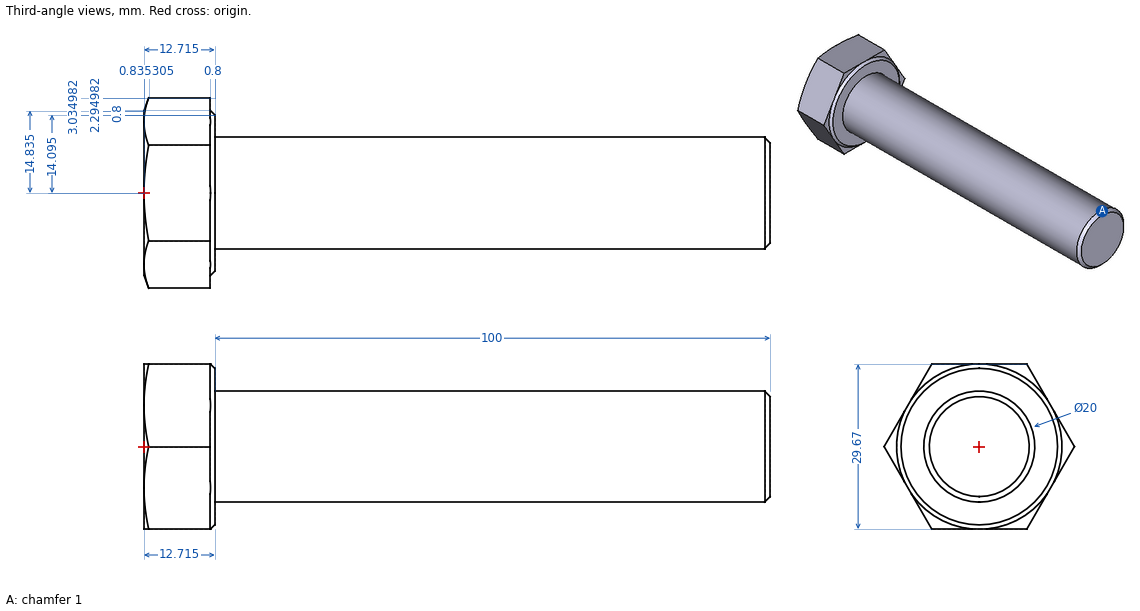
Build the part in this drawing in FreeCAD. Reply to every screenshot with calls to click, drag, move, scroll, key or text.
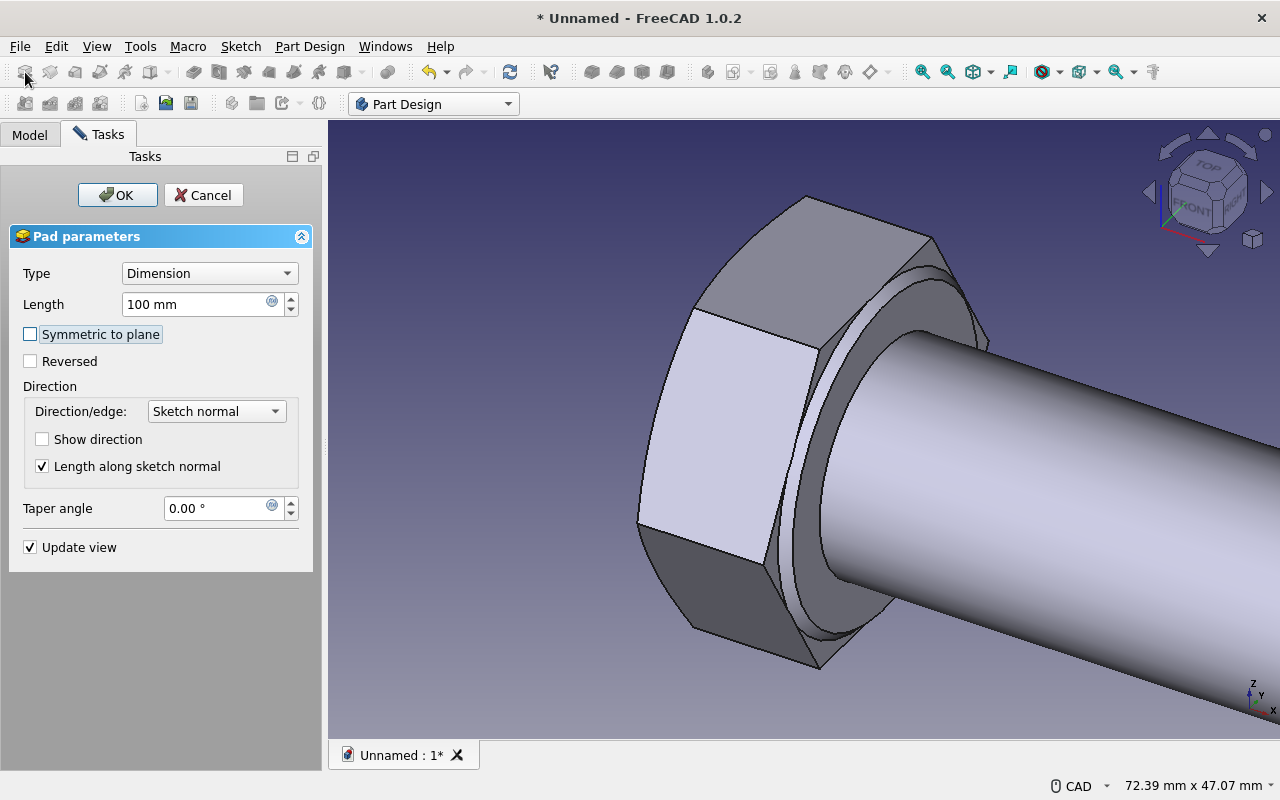
click(118, 195)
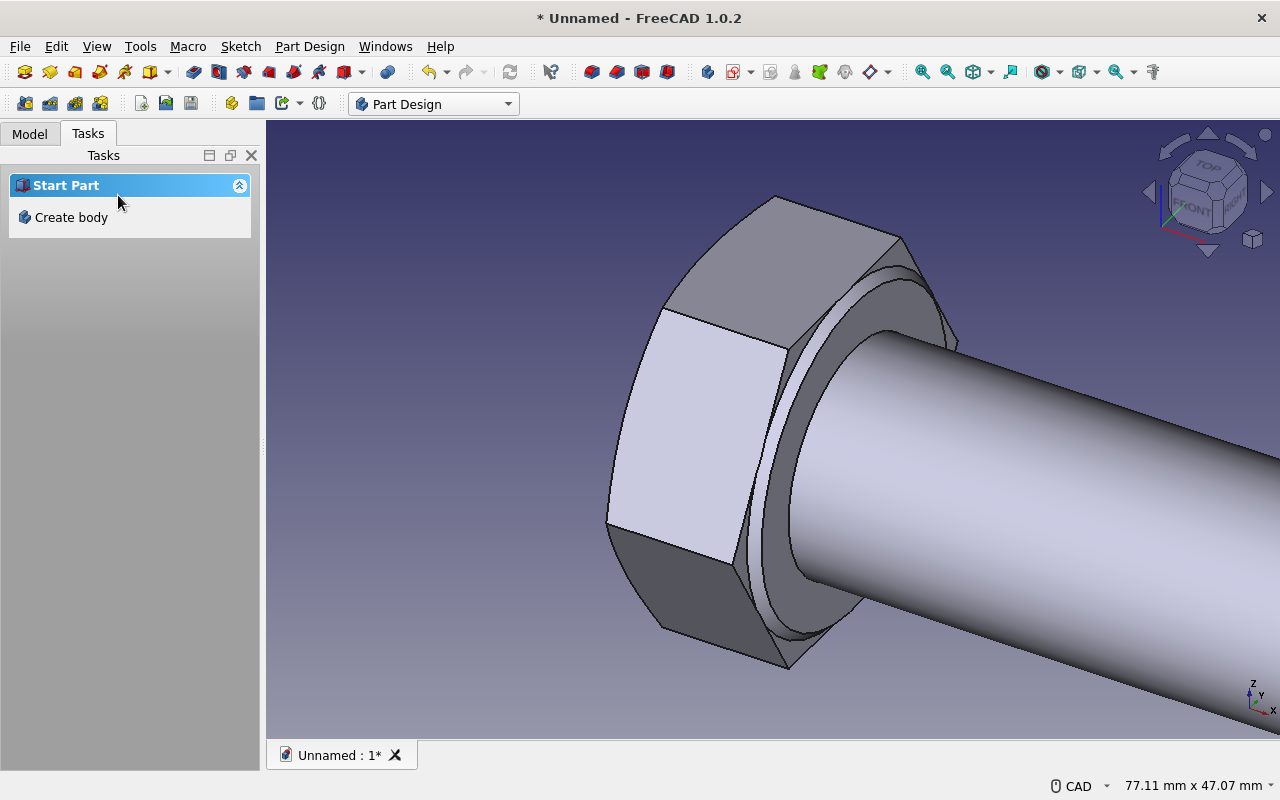
key(v)
key(f)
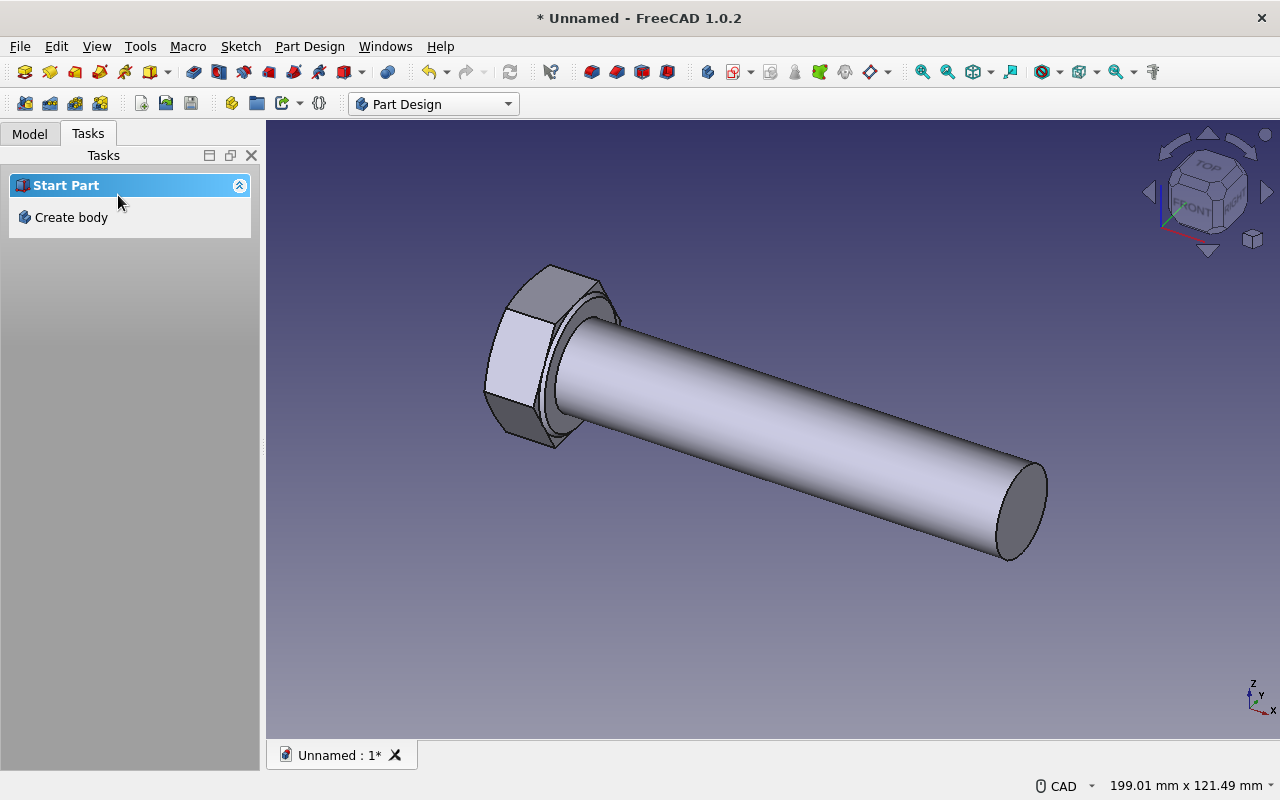
click(996, 536)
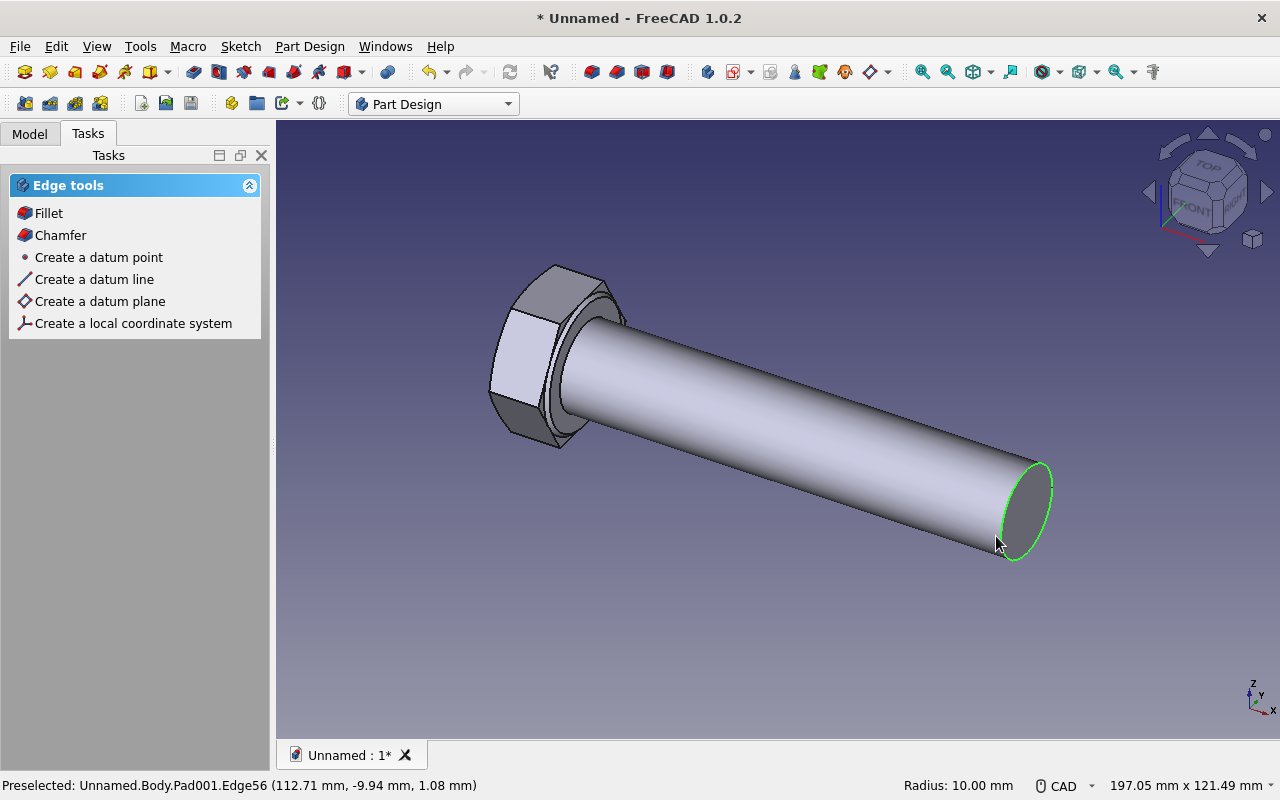
click(617, 72)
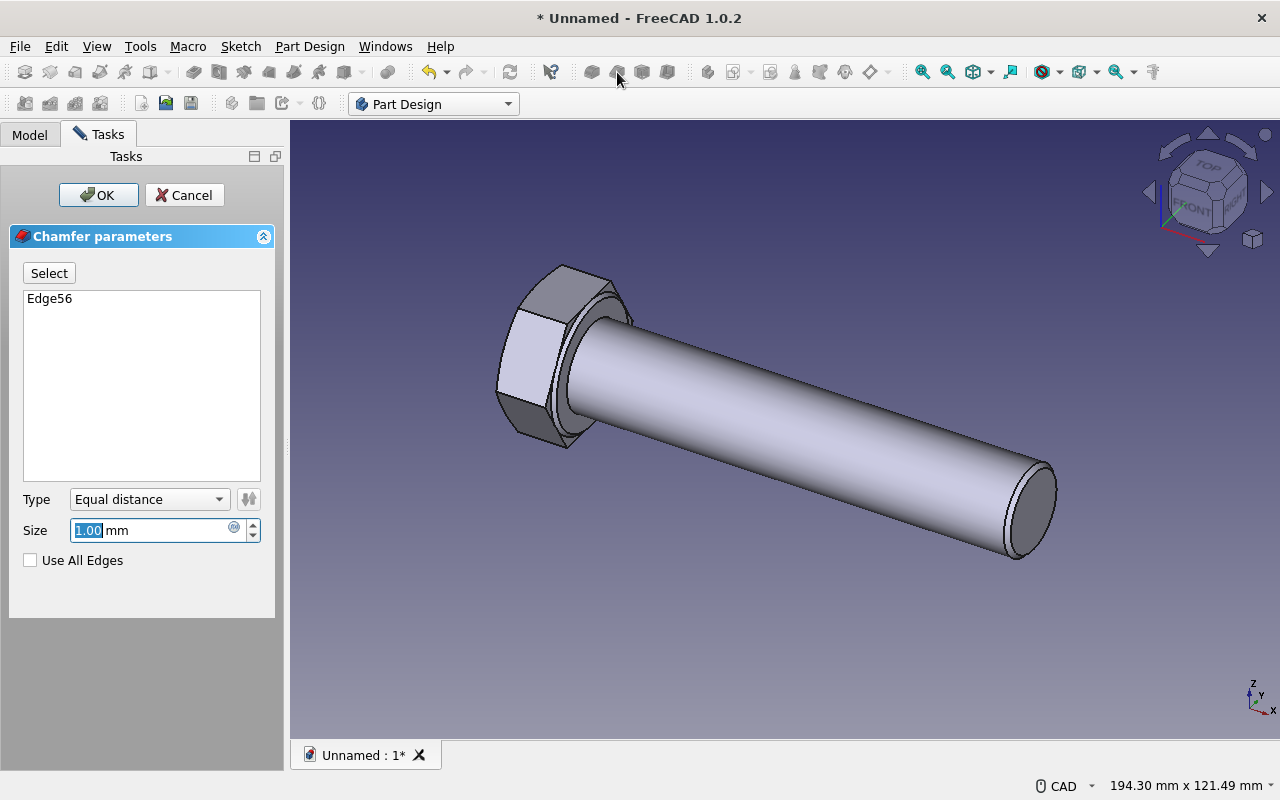
text(1)
key(Tab)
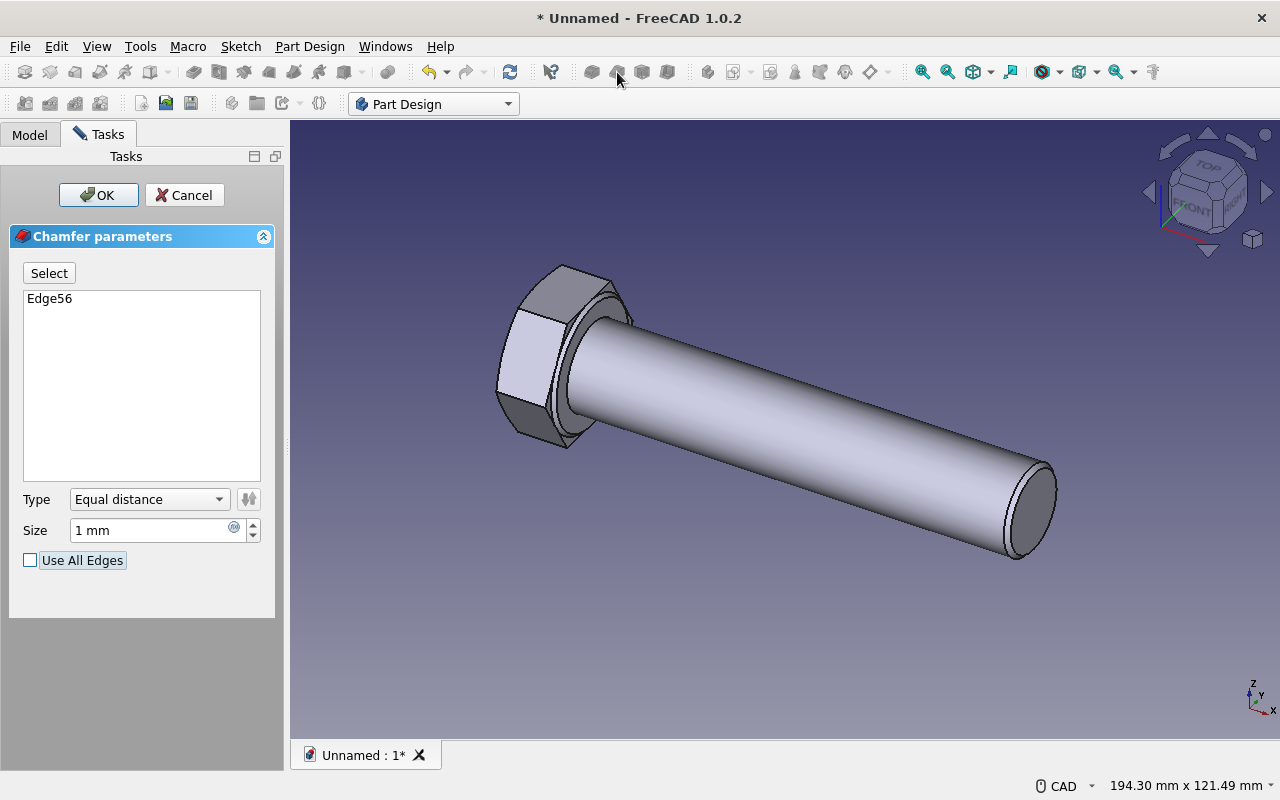
click(99, 195)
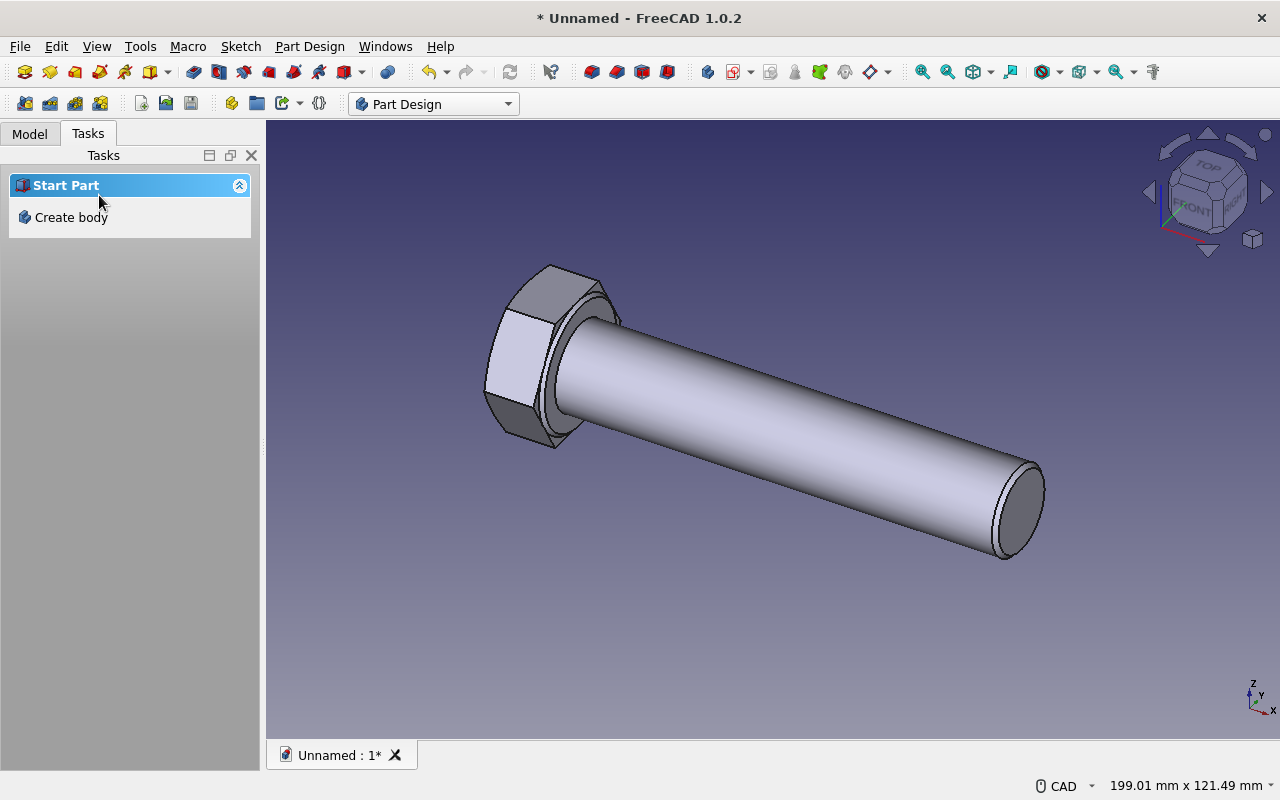
key(0)